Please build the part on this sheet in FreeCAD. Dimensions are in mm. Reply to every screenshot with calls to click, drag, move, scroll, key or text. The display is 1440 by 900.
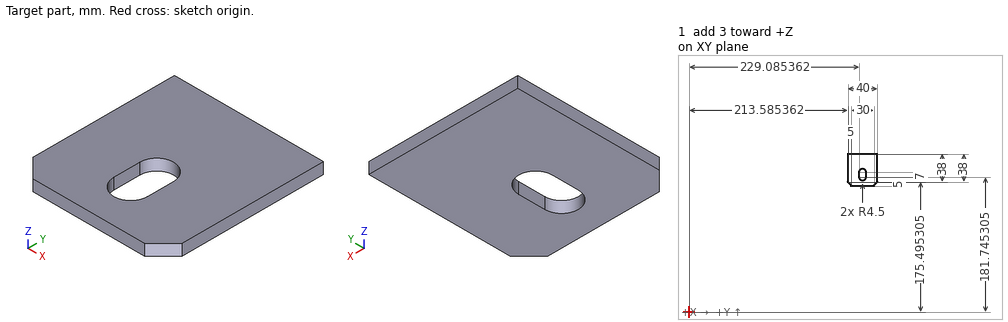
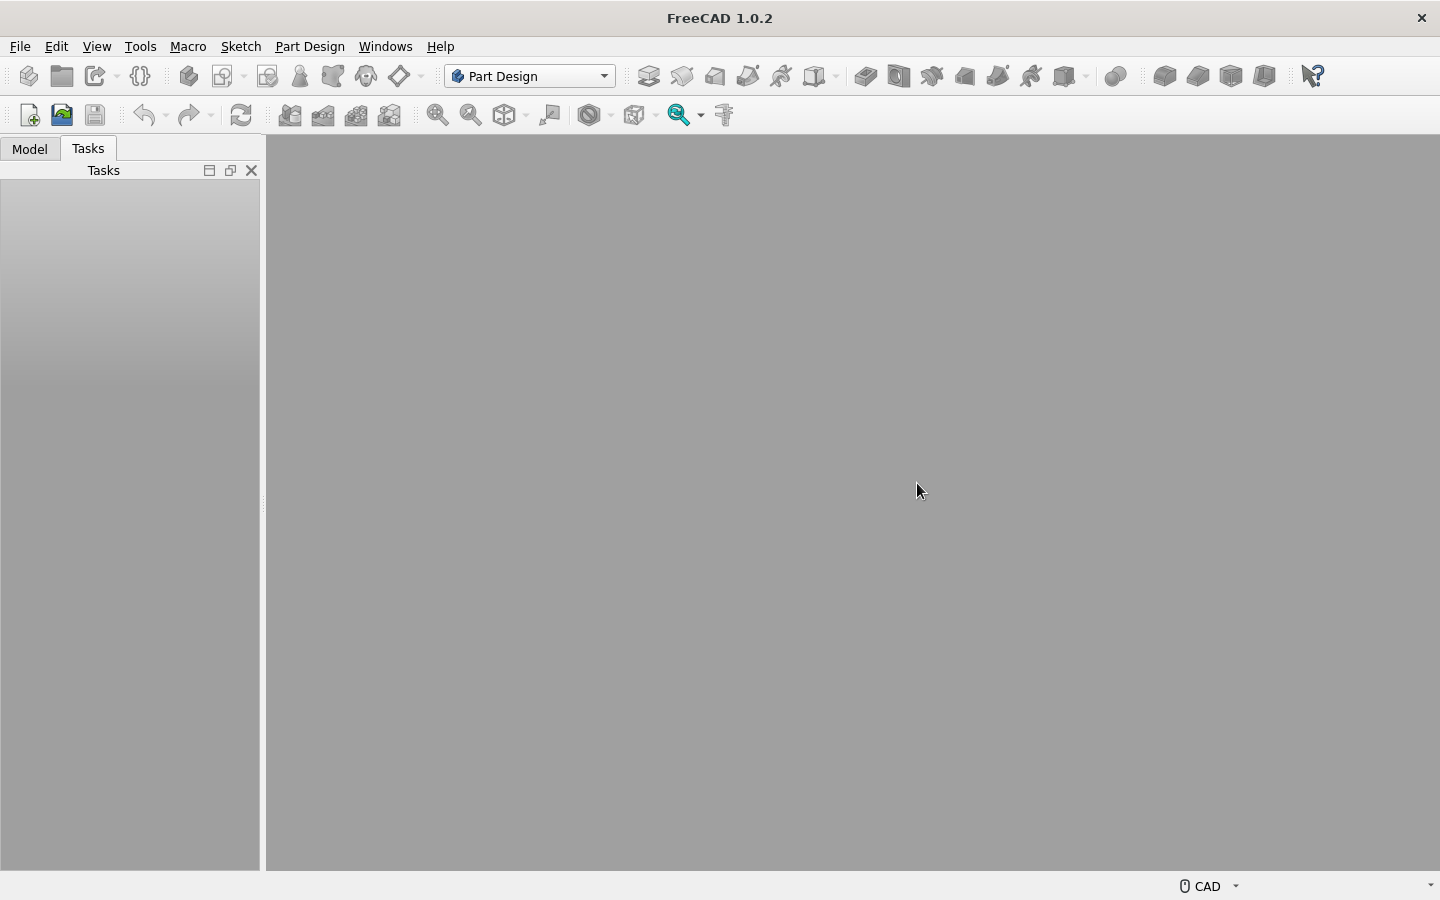
click(29, 116)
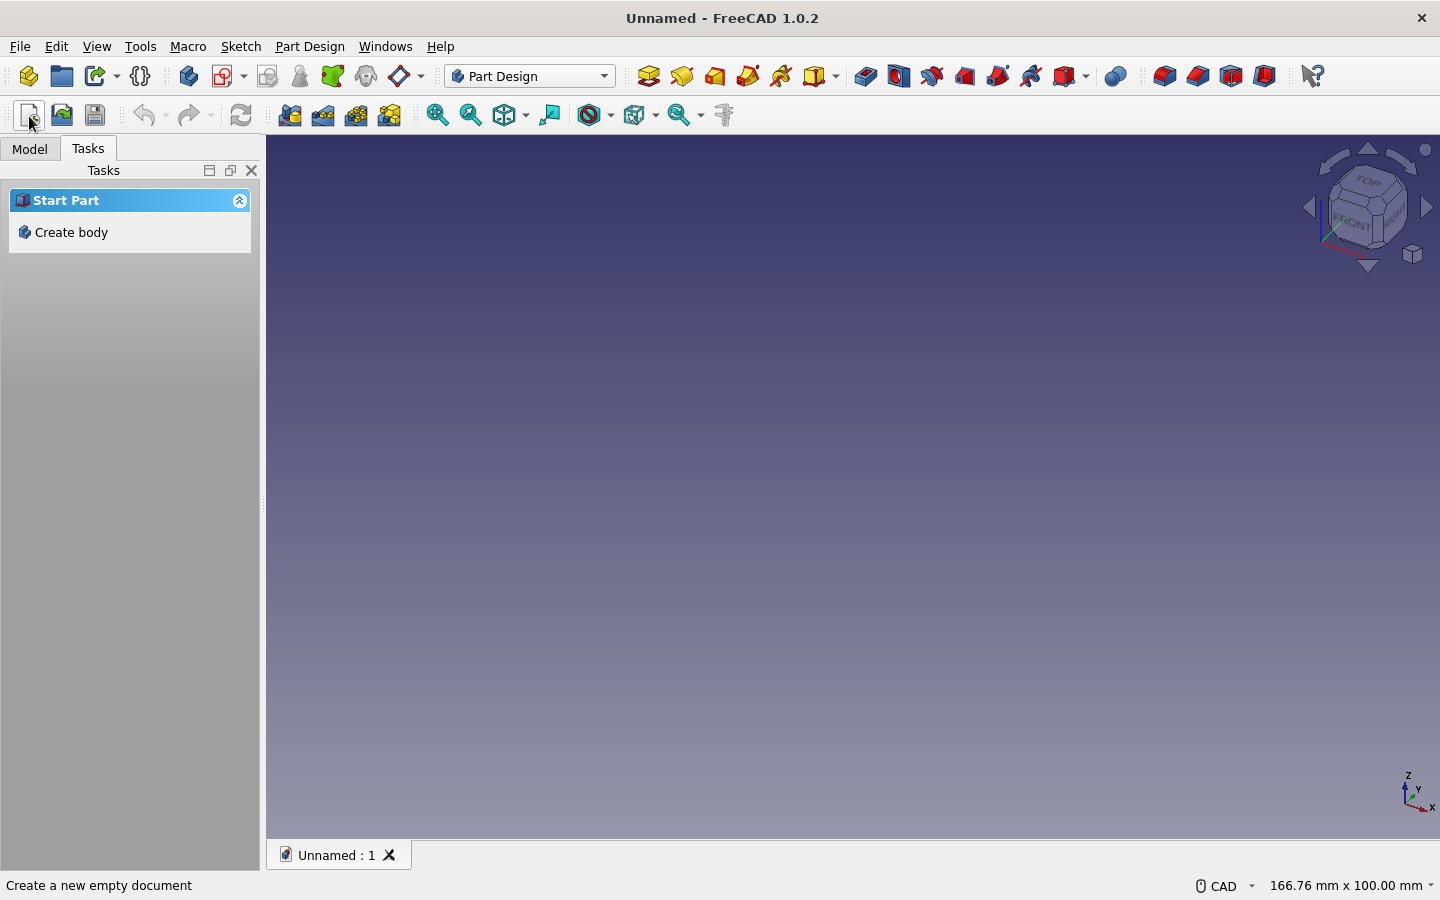
click(222, 76)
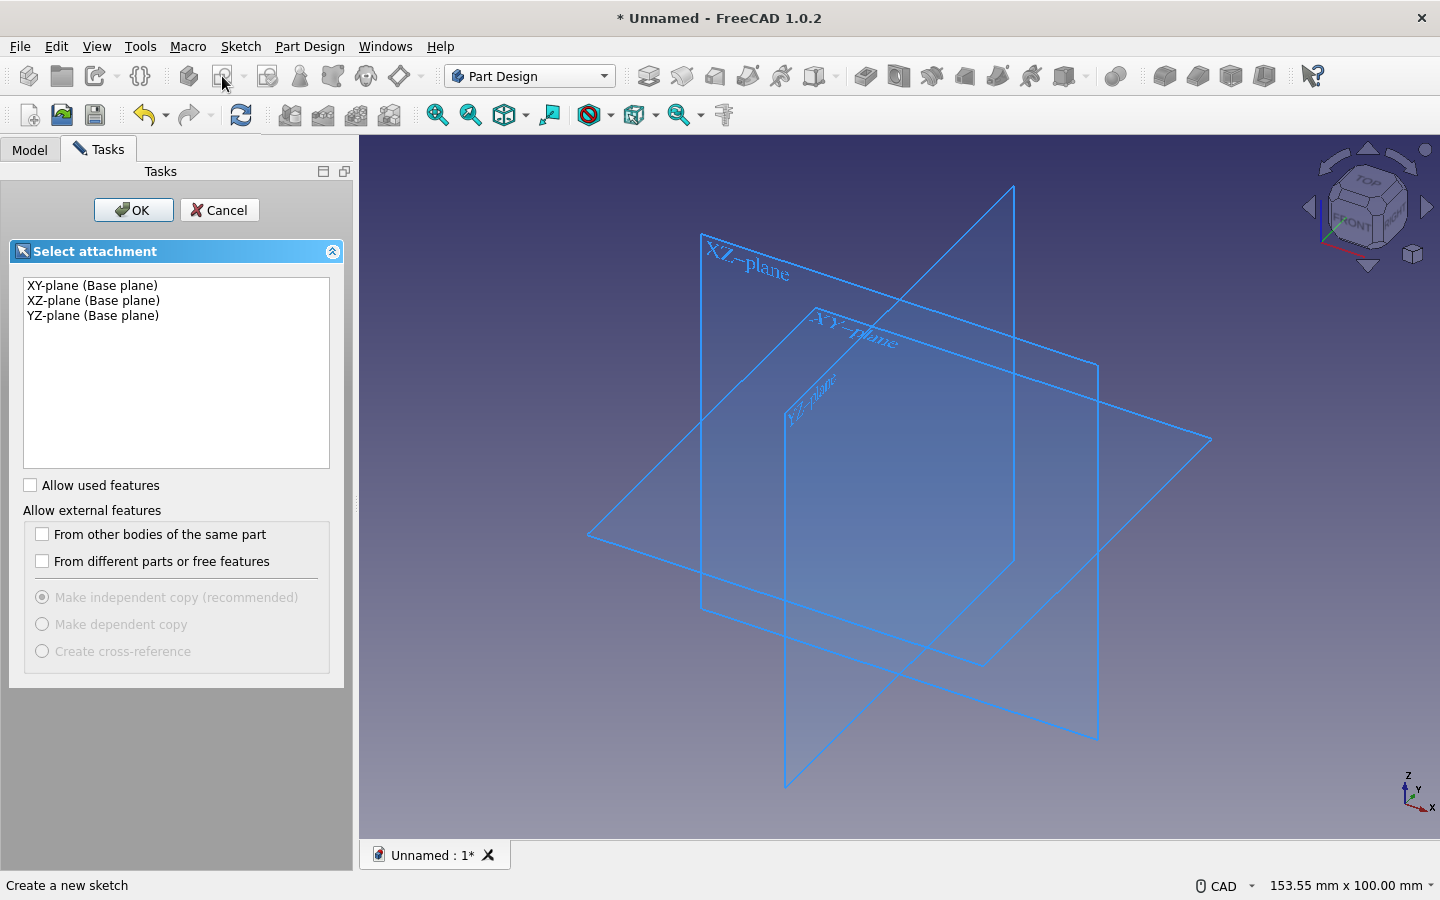
click(84, 286)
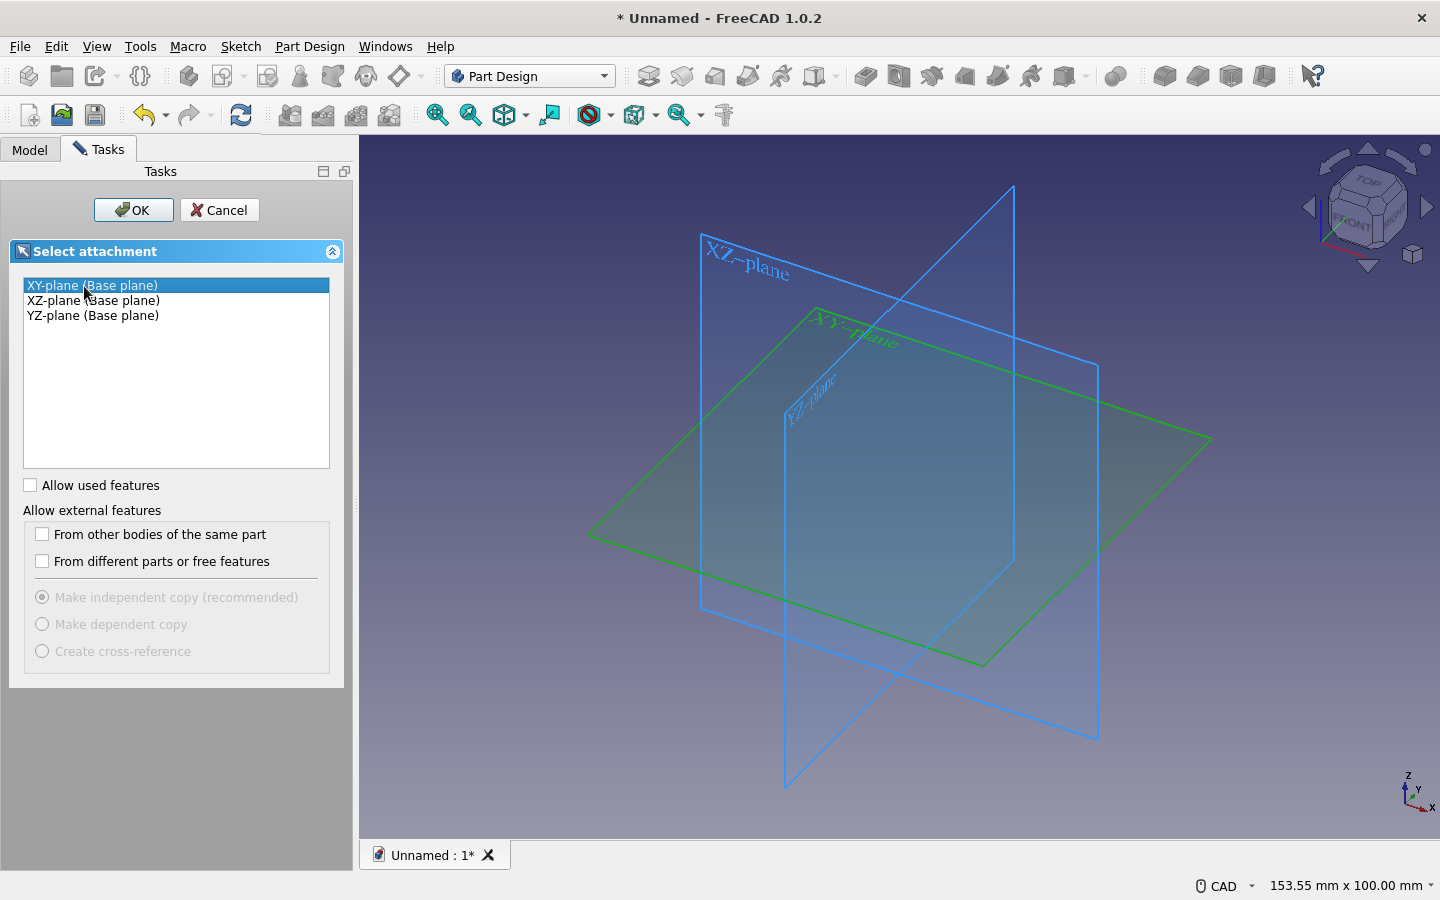
click(134, 210)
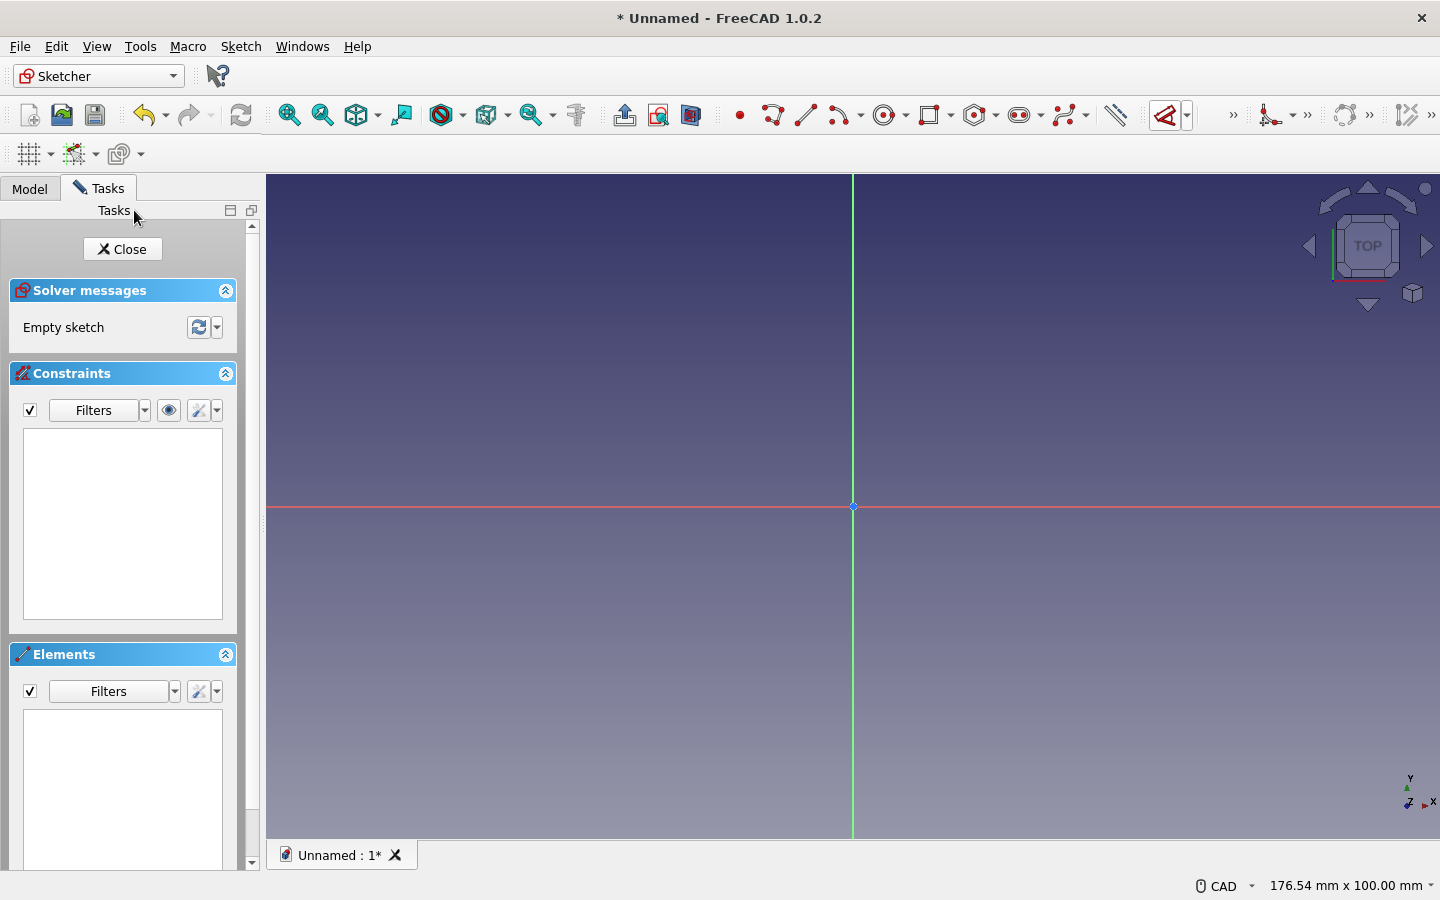
scroll(784, 506, down, 5)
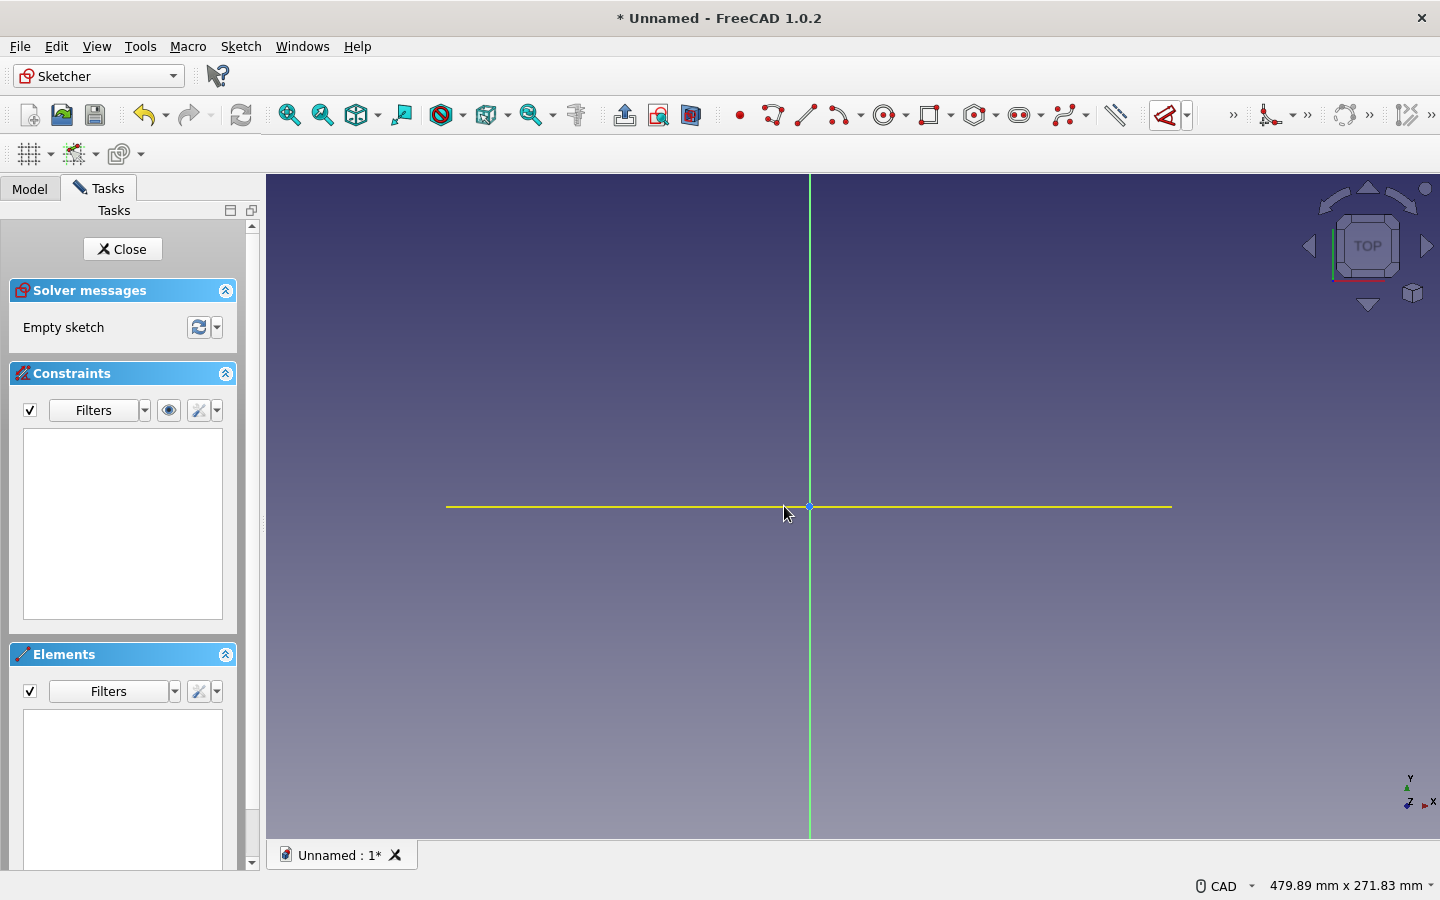
scroll(784, 506, down, 5)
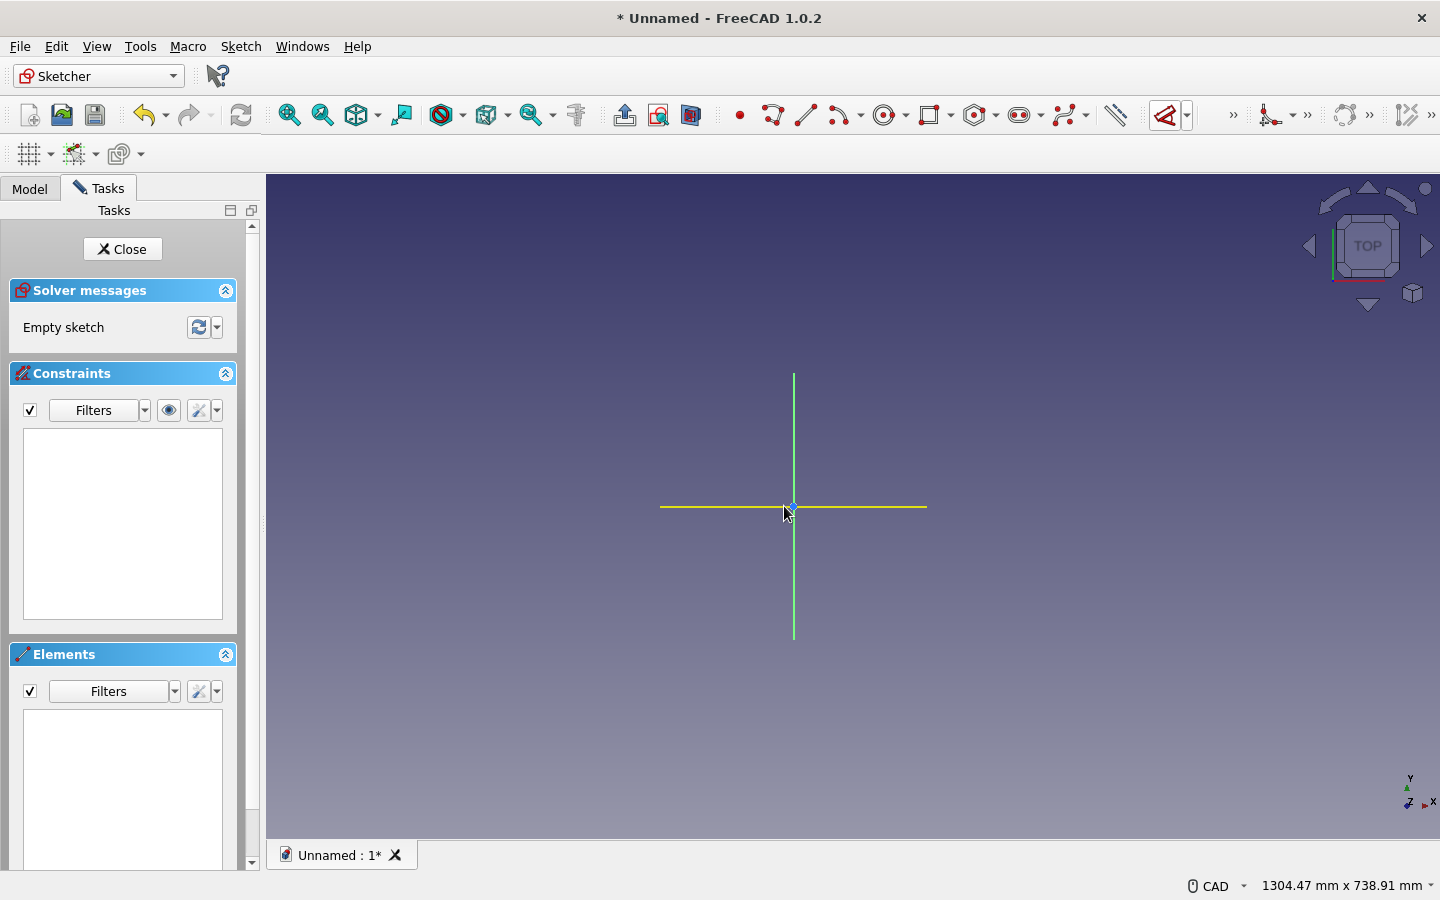
scroll(1026, 316, up, 12)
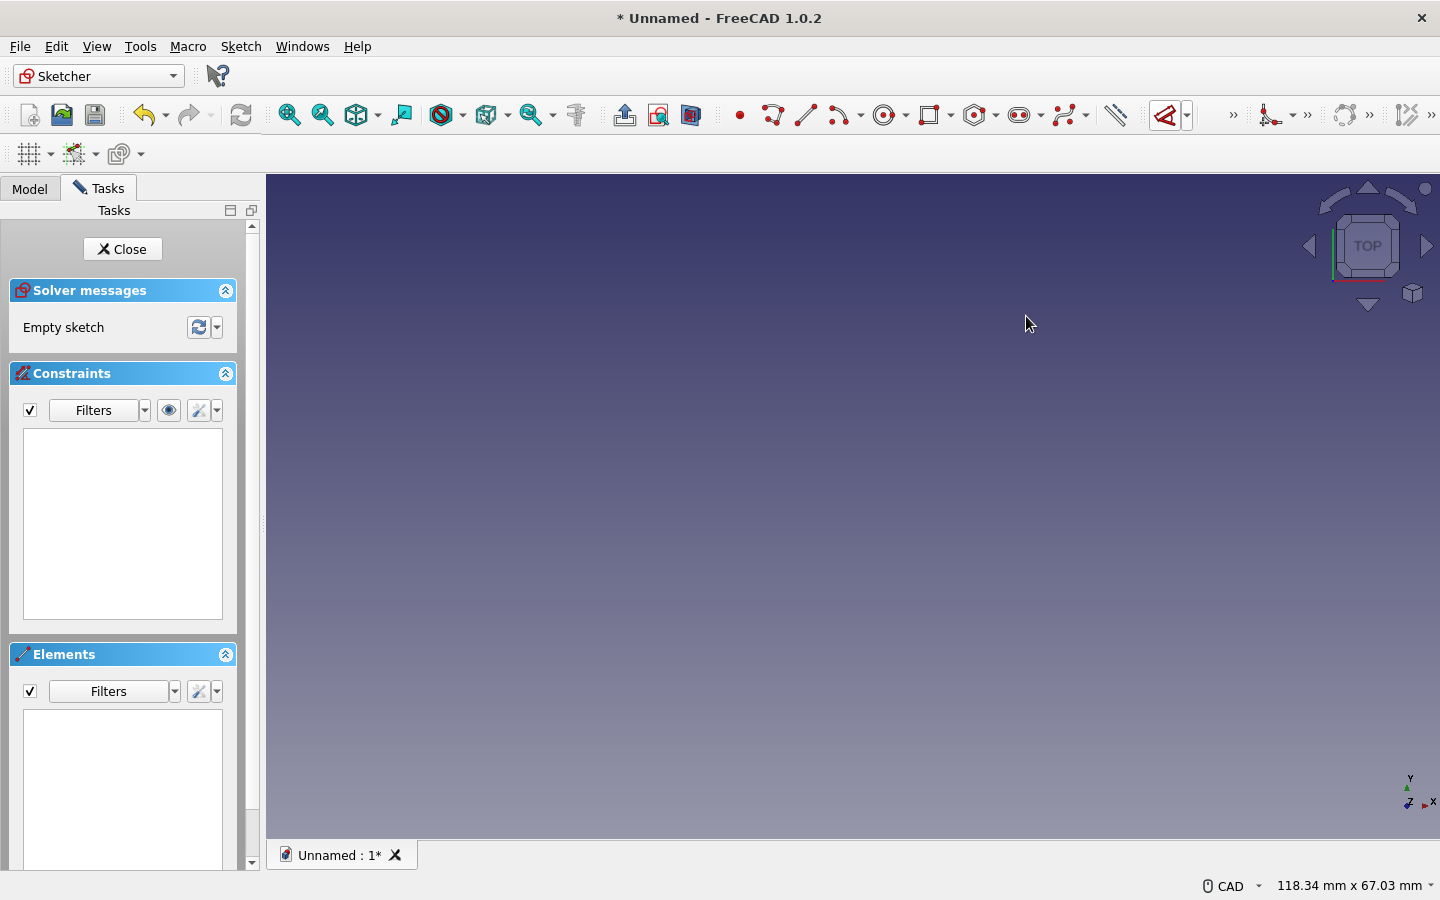
click(773, 116)